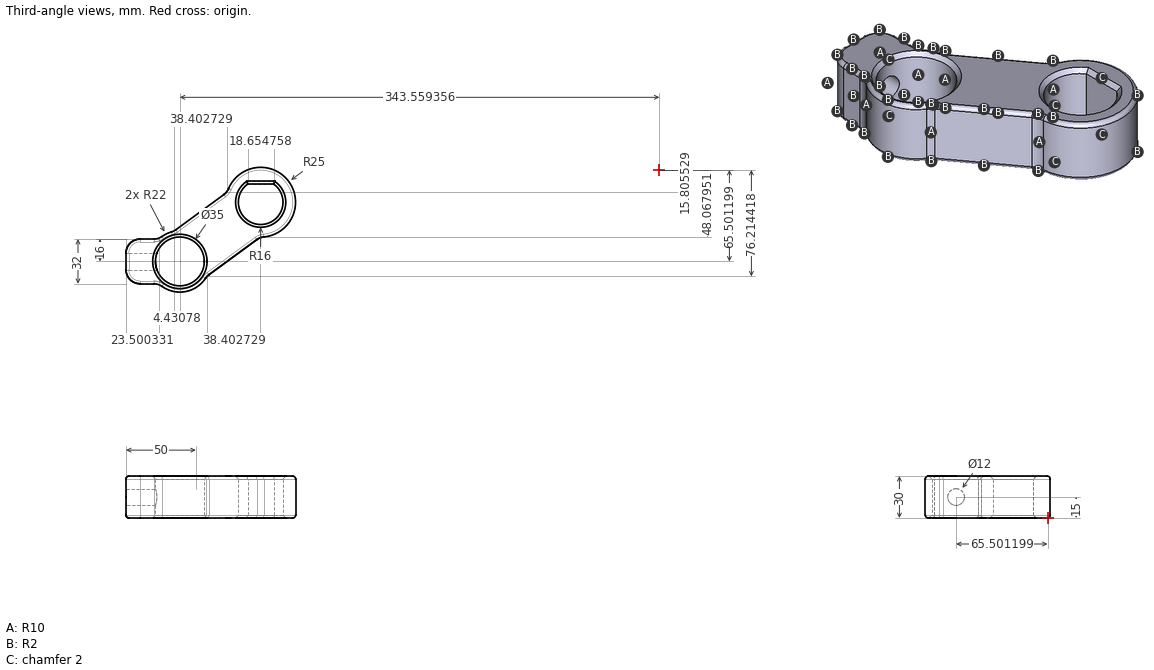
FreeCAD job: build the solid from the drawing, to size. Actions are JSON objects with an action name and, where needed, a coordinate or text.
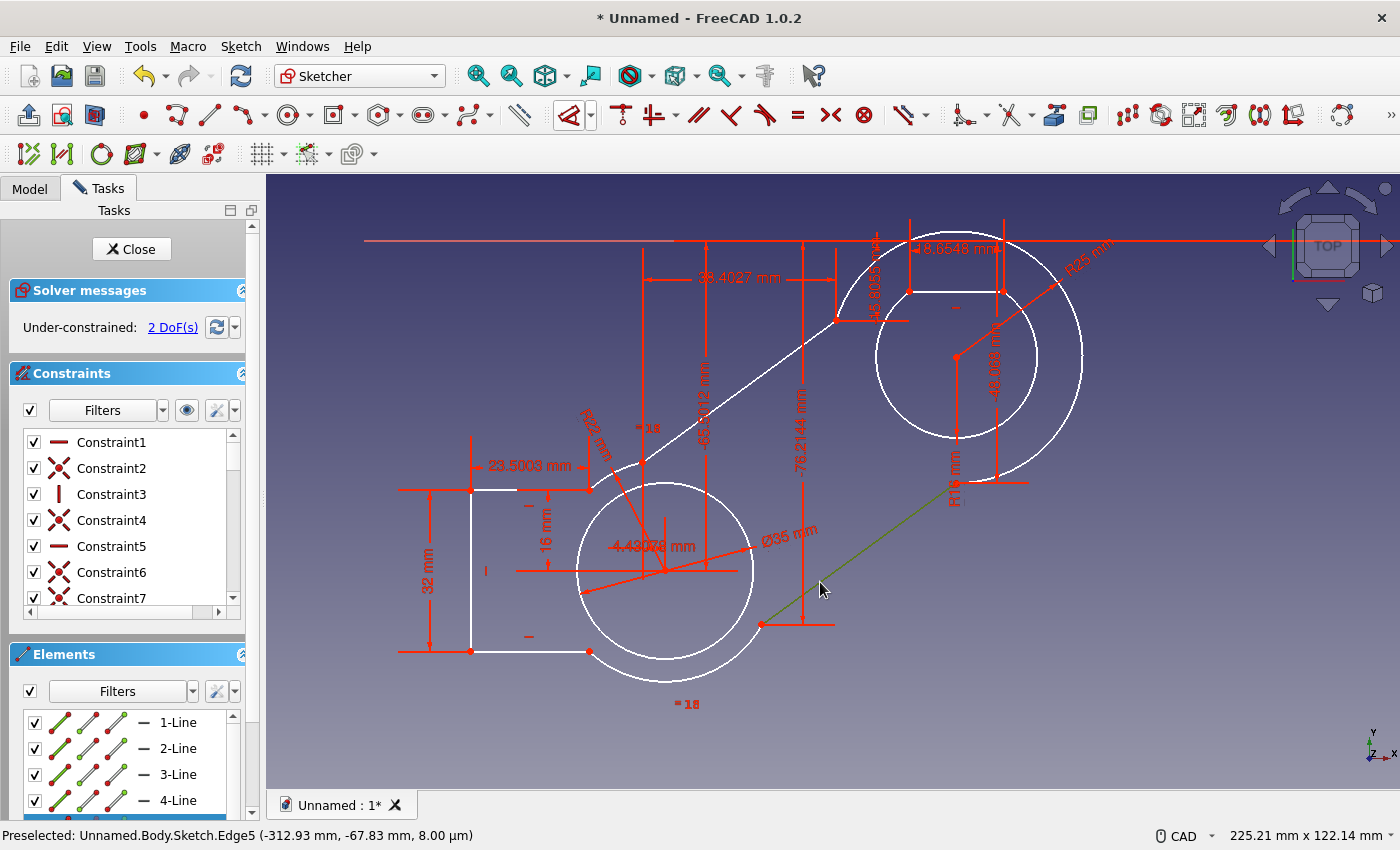
{"action": "key", "text": "l"}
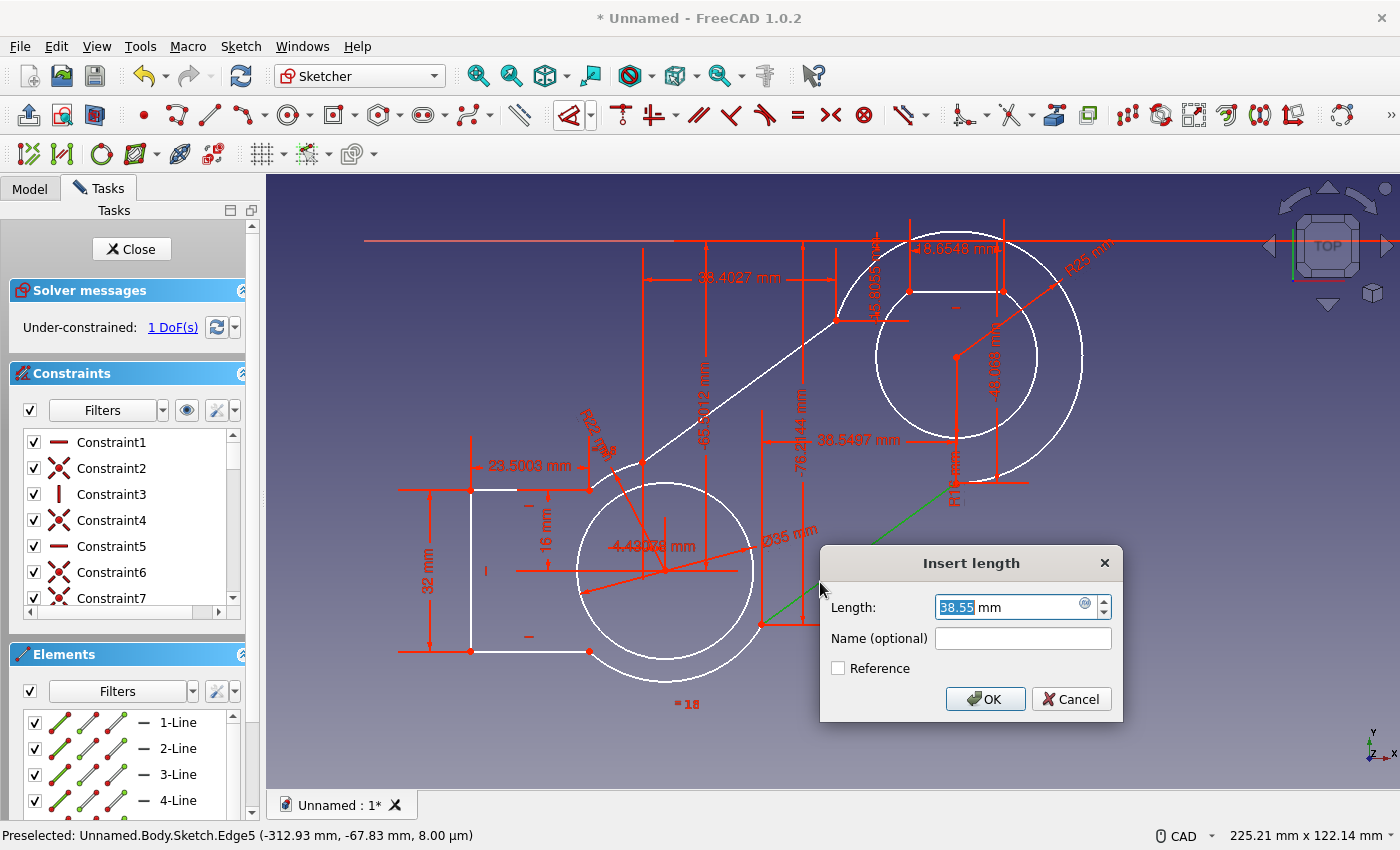
{"action": "type", "text": "38.402729"}
{"action": "key", "text": "Return"}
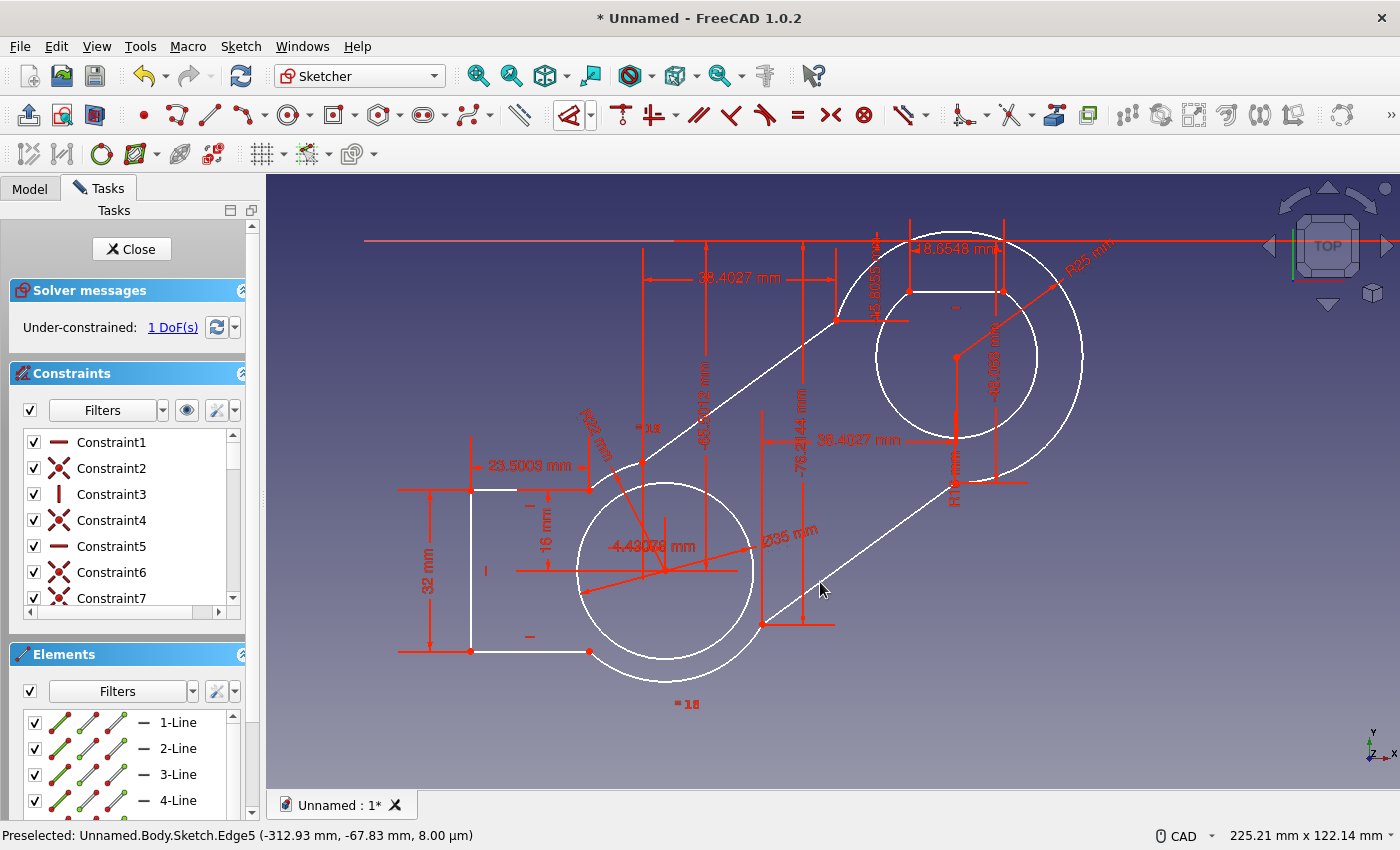
{"action": "left_click", "coordinate": [665, 571]}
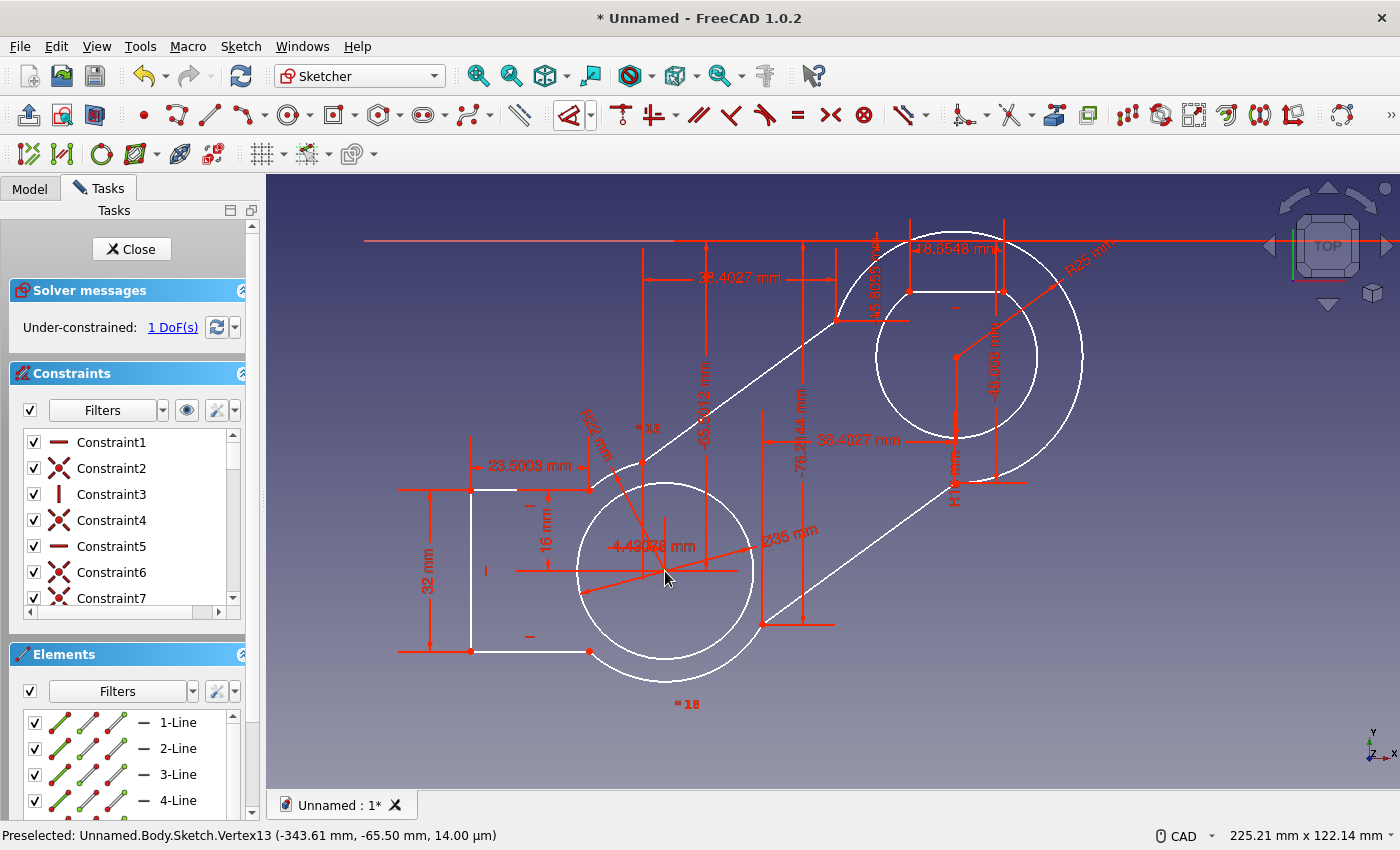
{"action": "left_click", "coordinate": [590, 116]}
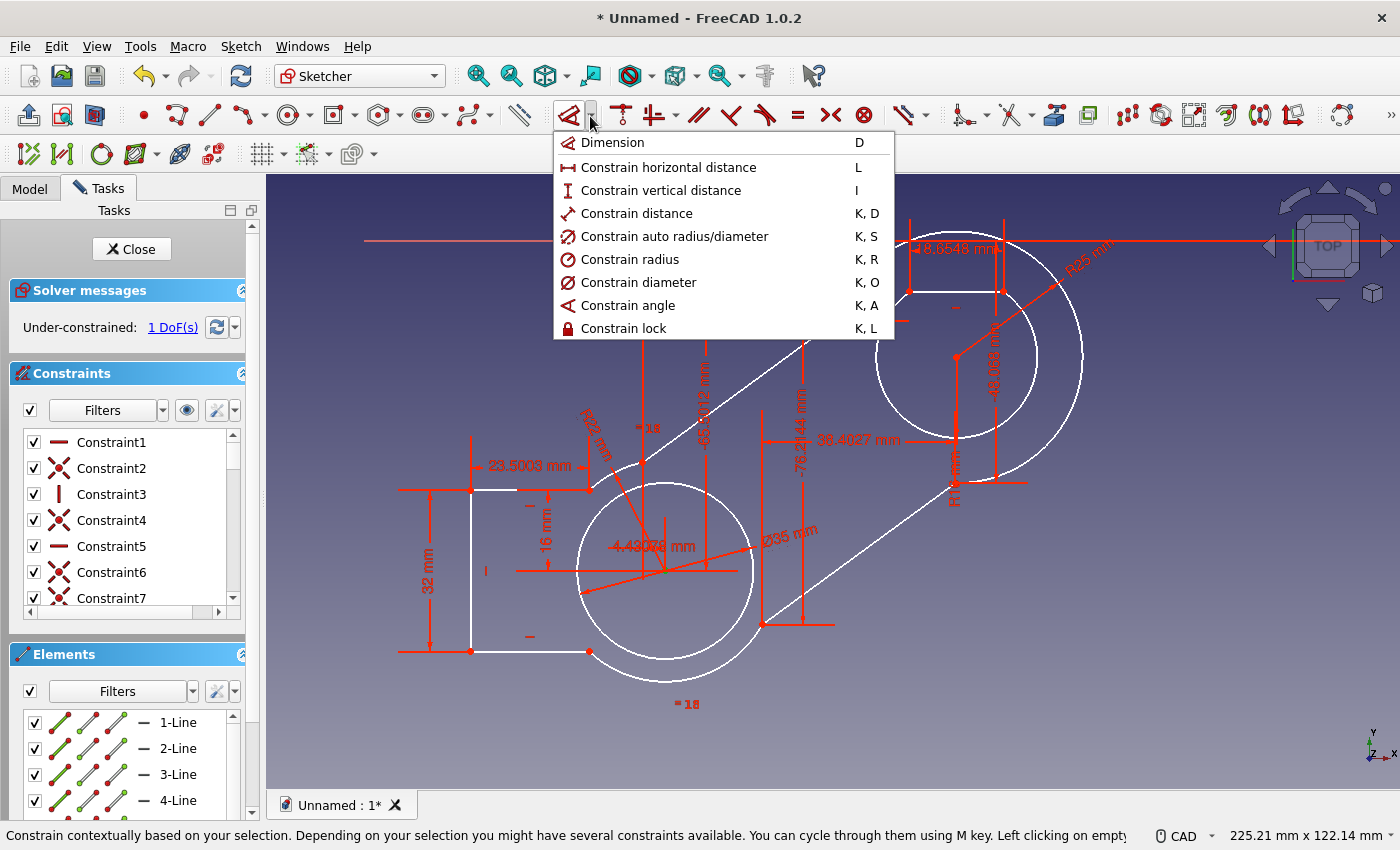
{"action": "left_click", "coordinate": [724, 168]}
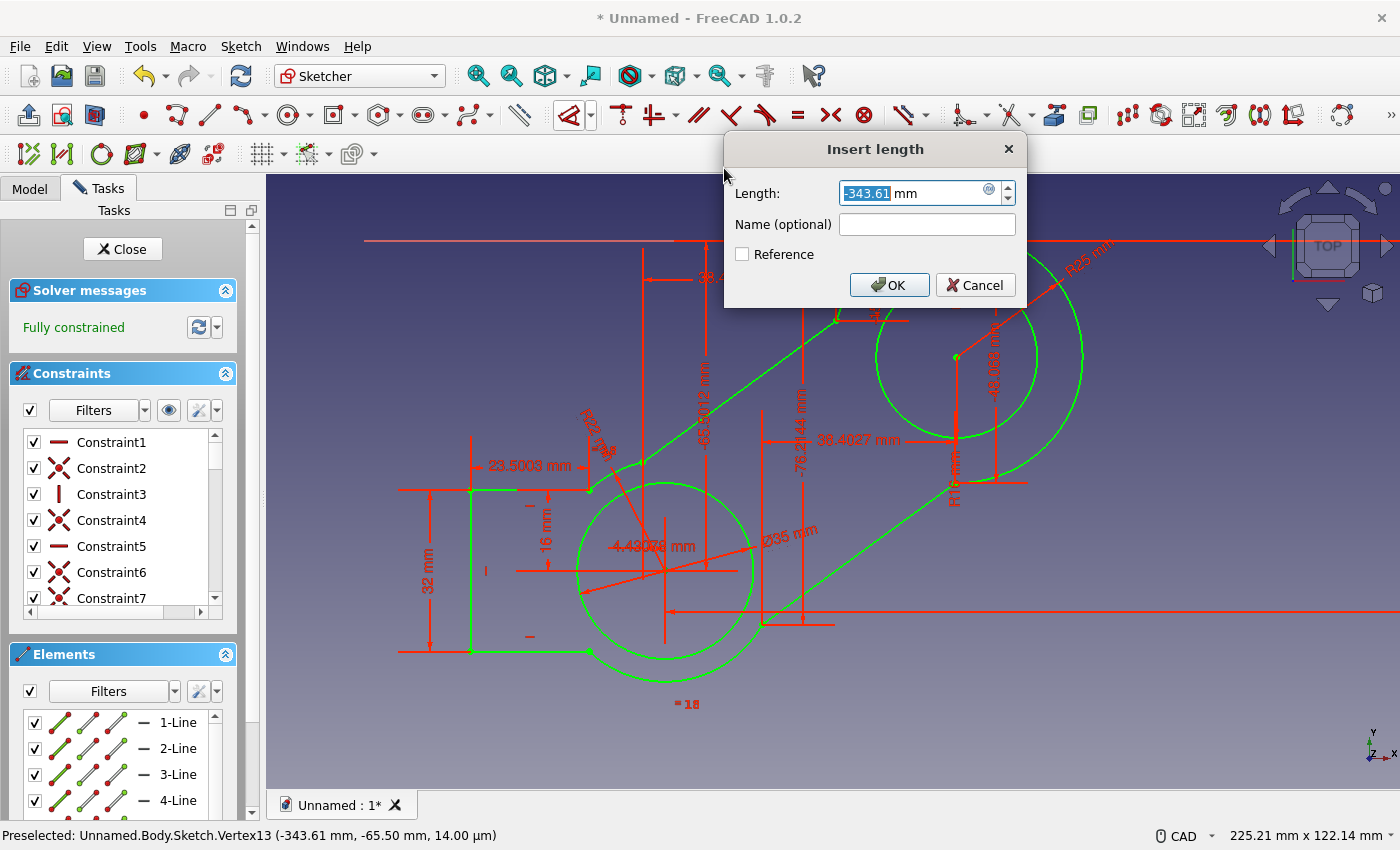
{"action": "type", "text": "-343.559356"}
{"action": "key", "text": "Return"}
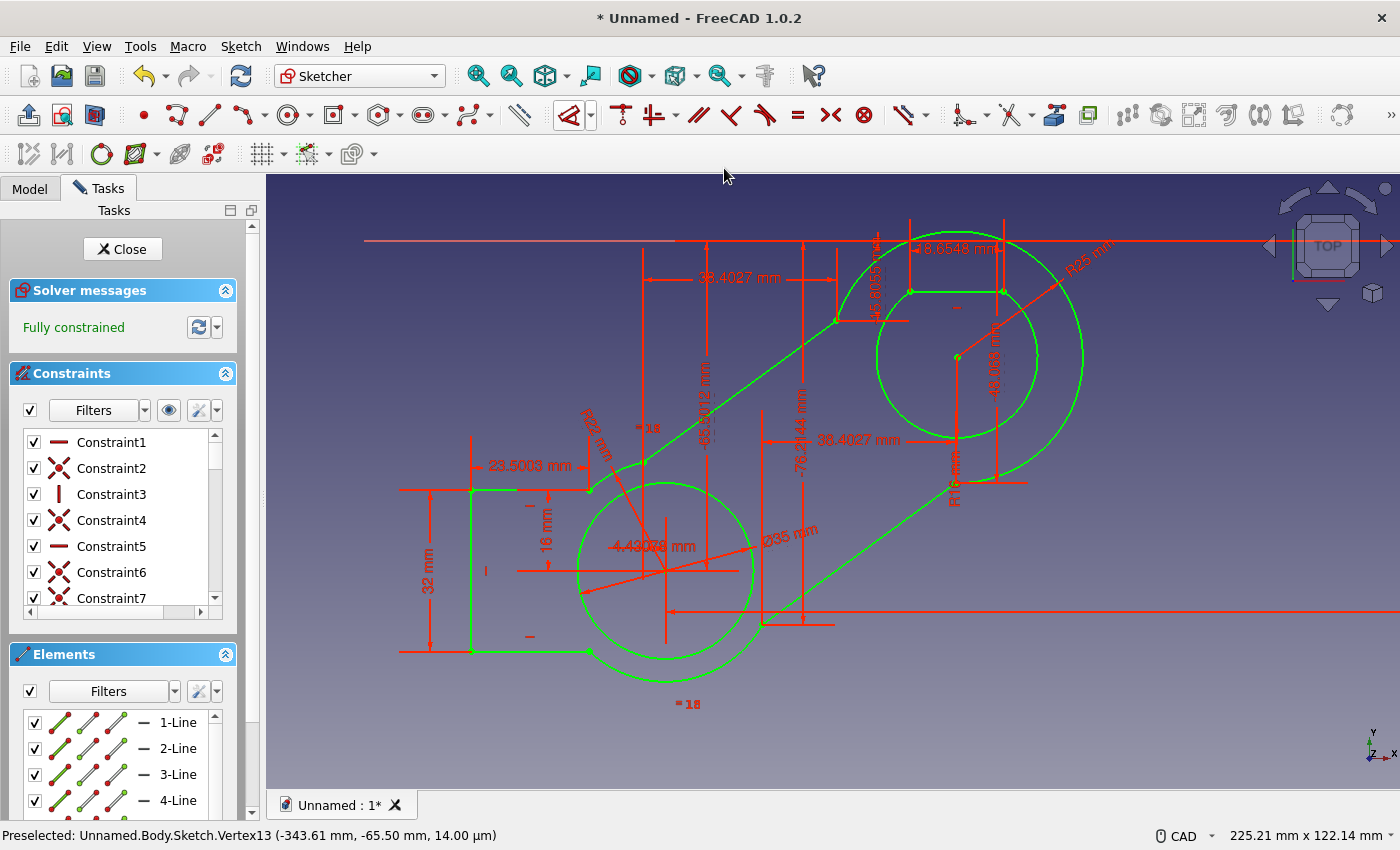
{"action": "left_click", "coordinate": [123, 249]}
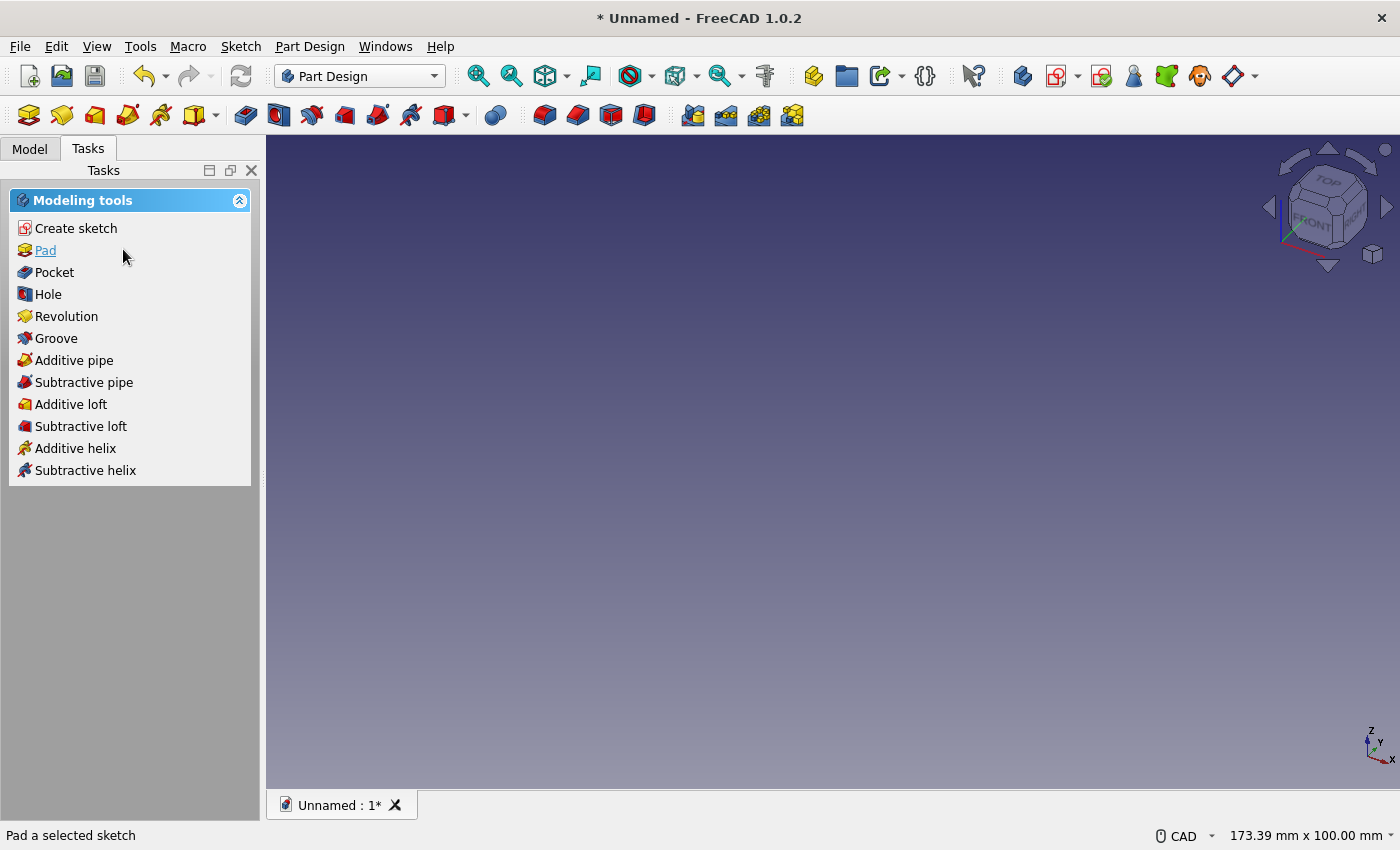
{"action": "left_click", "coordinate": [29, 116]}